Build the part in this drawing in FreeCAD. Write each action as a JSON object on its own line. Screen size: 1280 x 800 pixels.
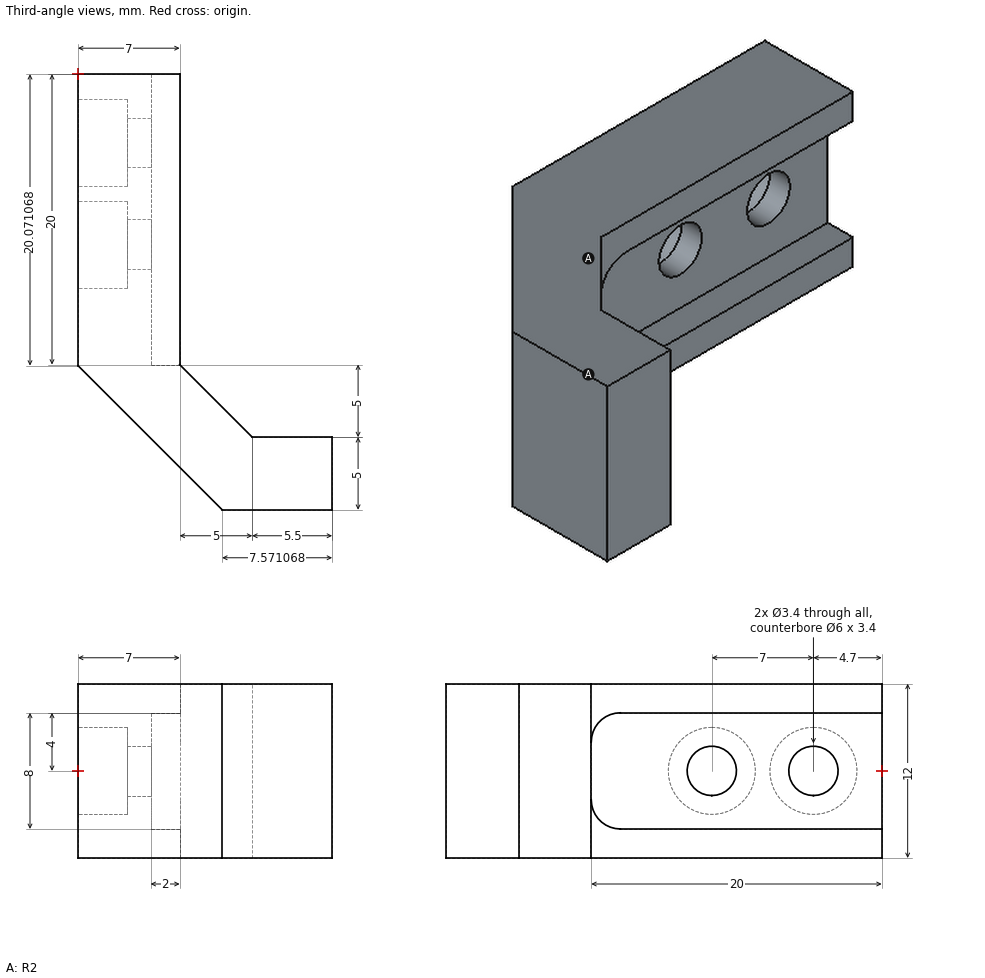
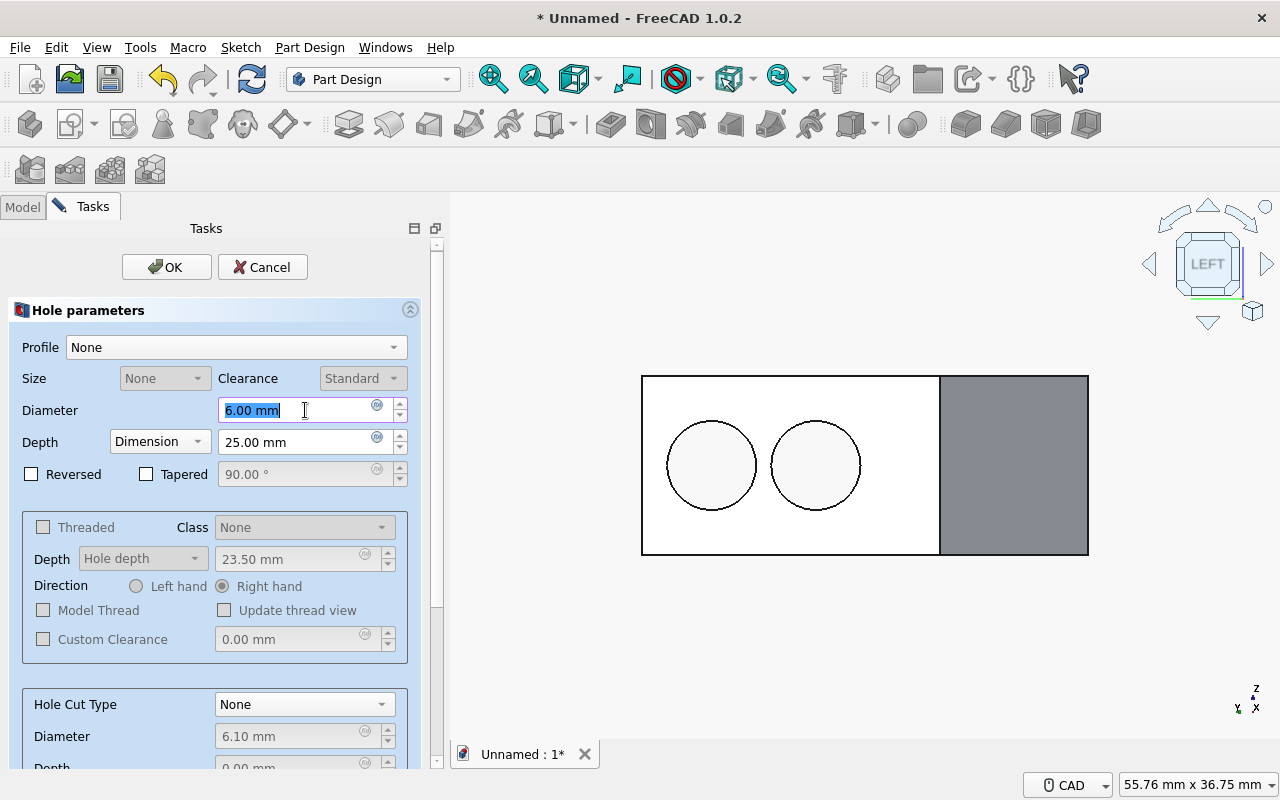
{"action": "type", "text": "3.4"}
{"action": "key", "text": "Tab"}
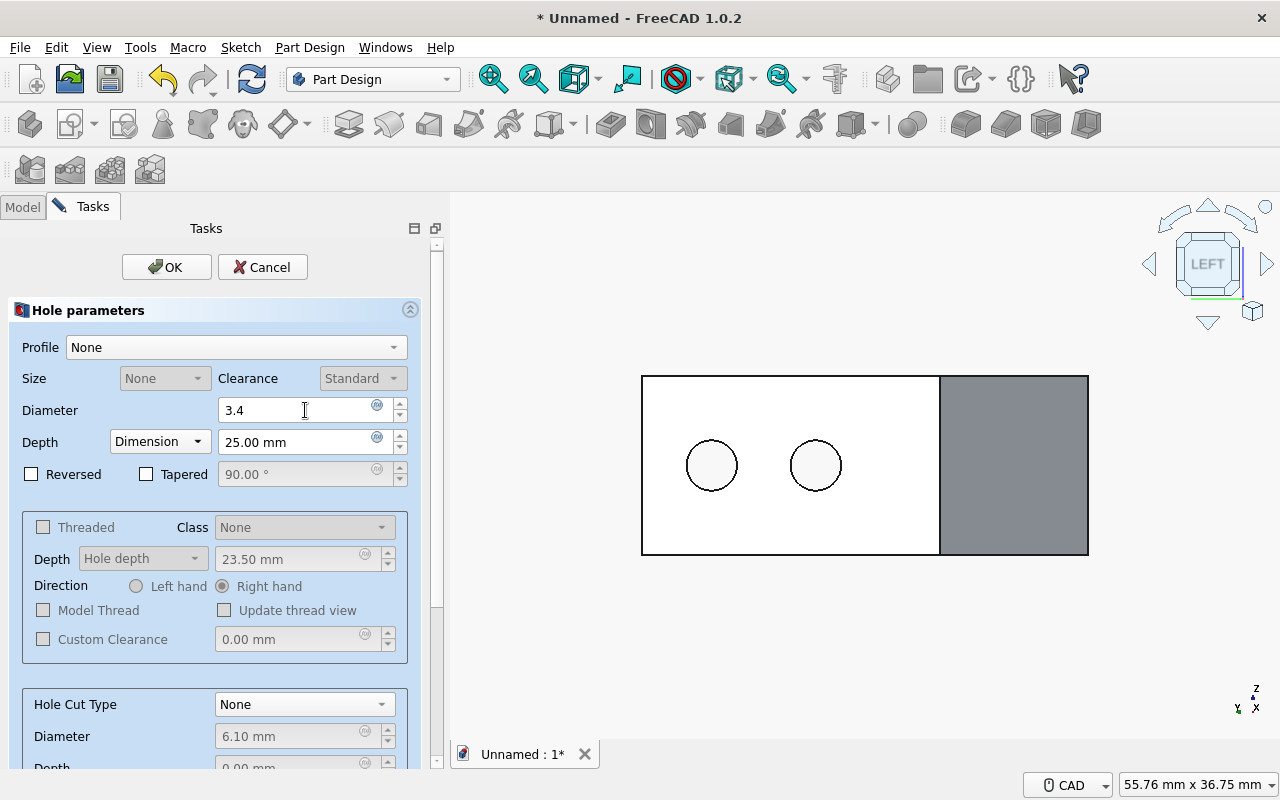
{"action": "left_click", "coordinate": [161, 442]}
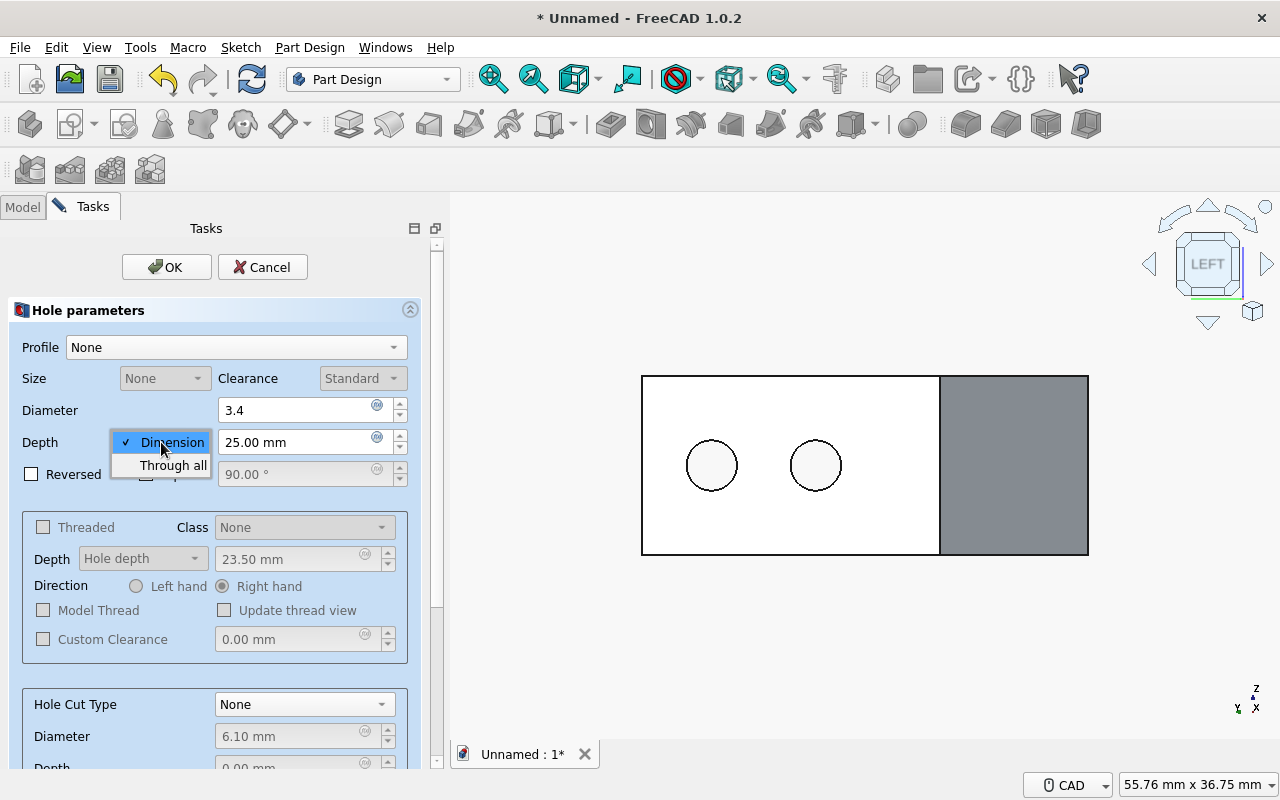
{"action": "left_click", "coordinate": [160, 466]}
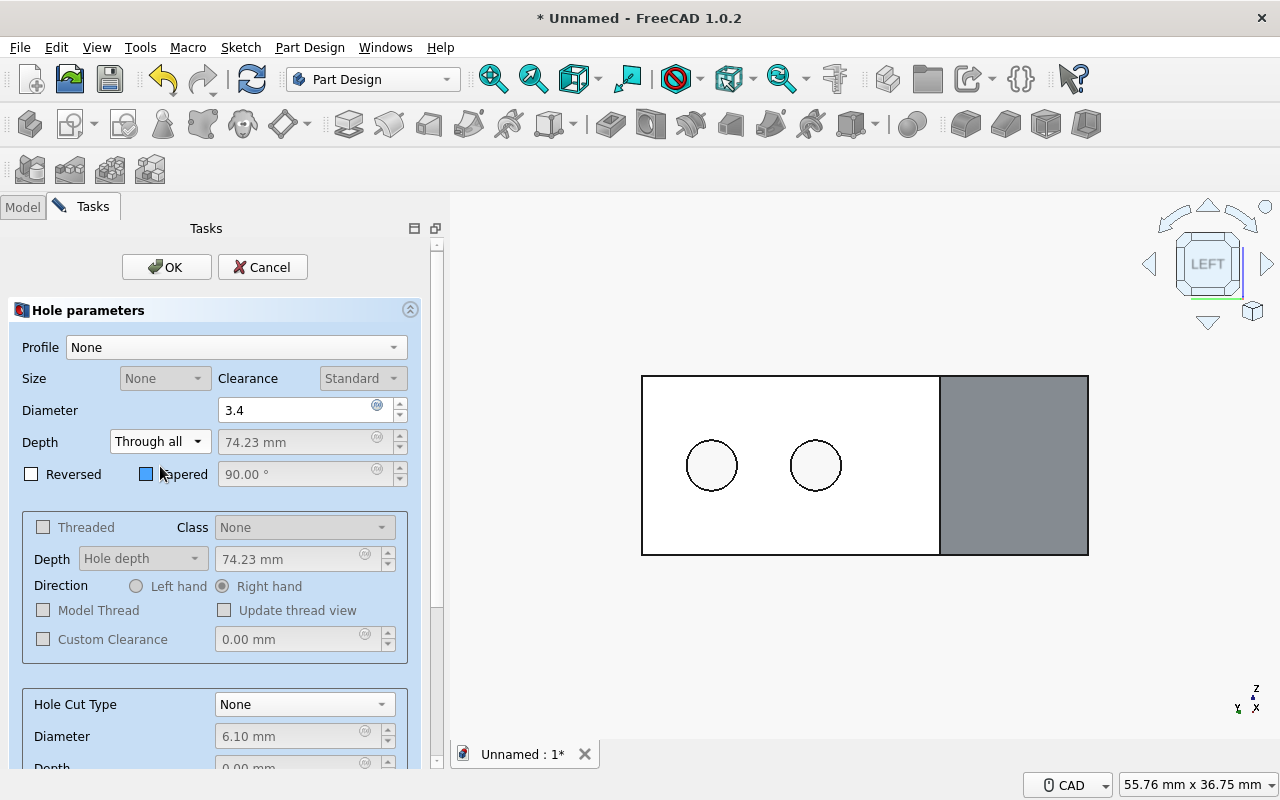
{"action": "left_click", "coordinate": [306, 704]}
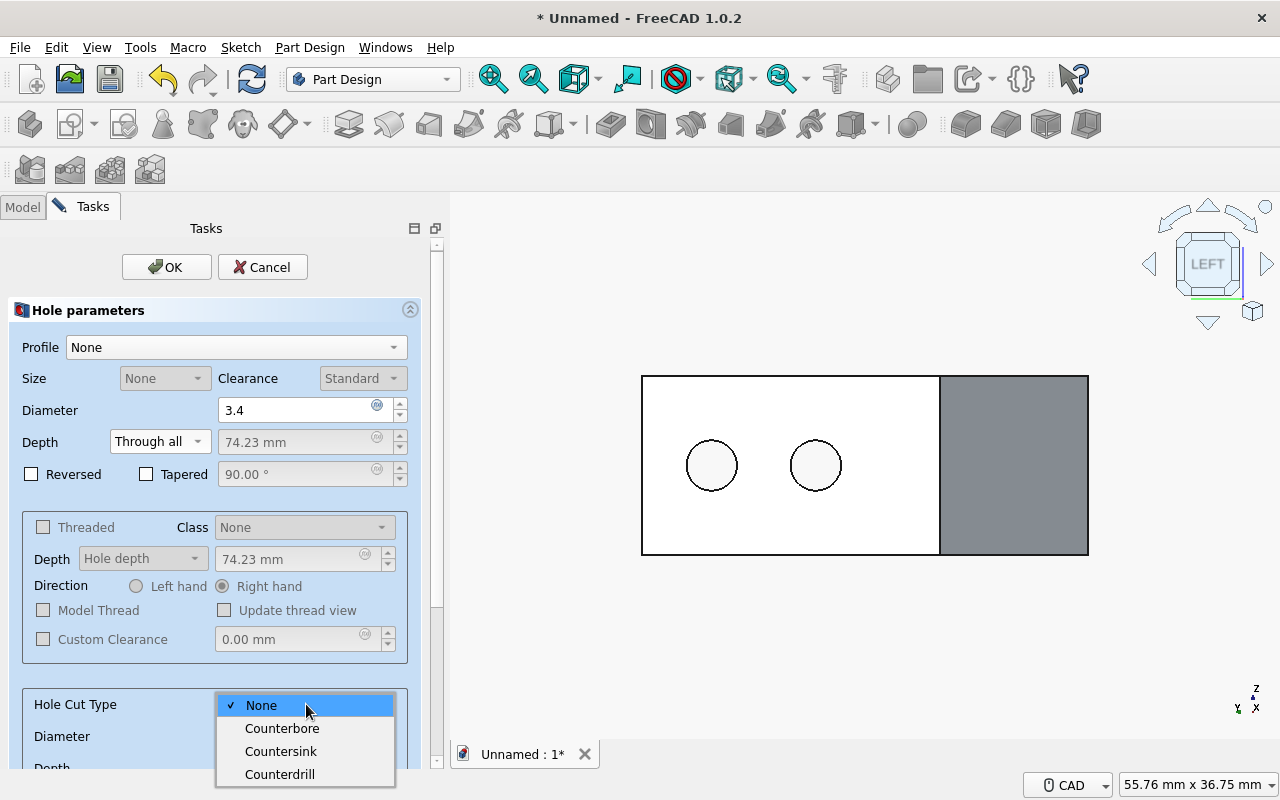
{"action": "left_click", "coordinate": [304, 728]}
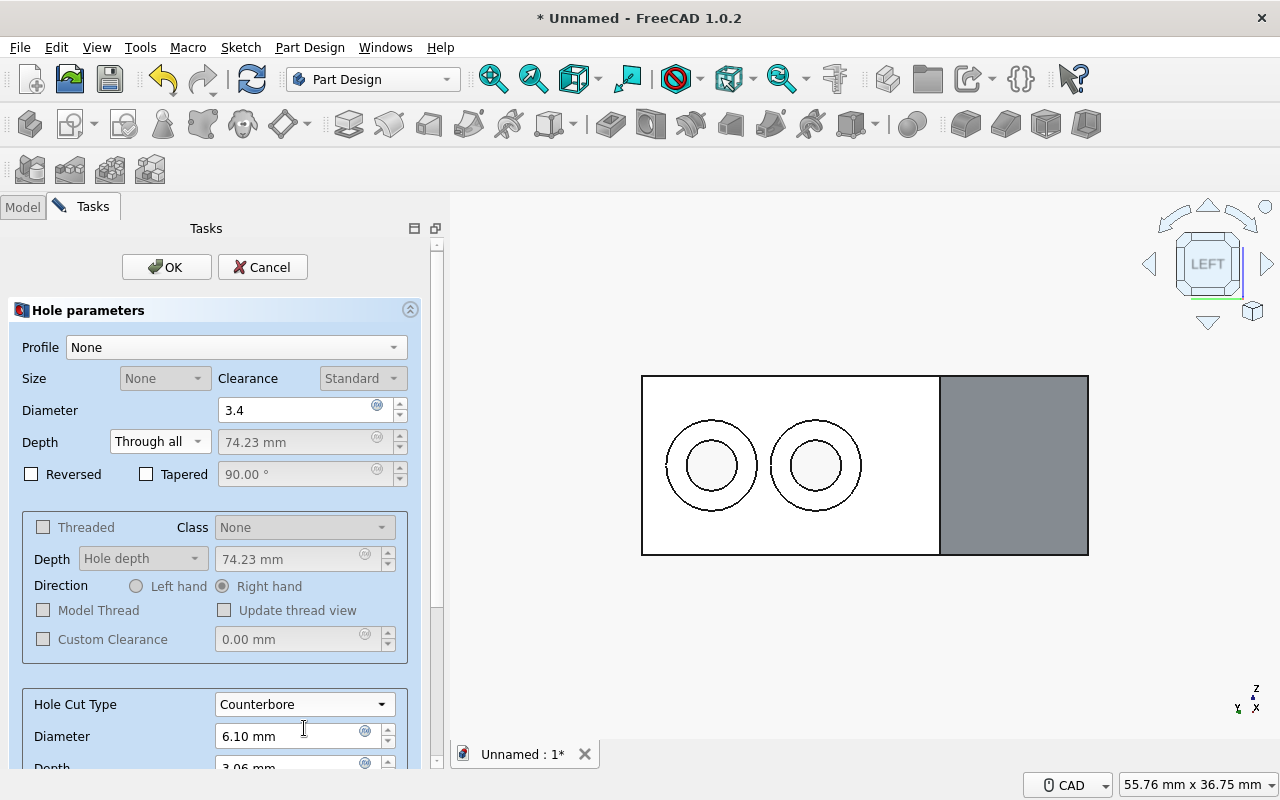
{"action": "triple_click", "coordinate": [298, 736]}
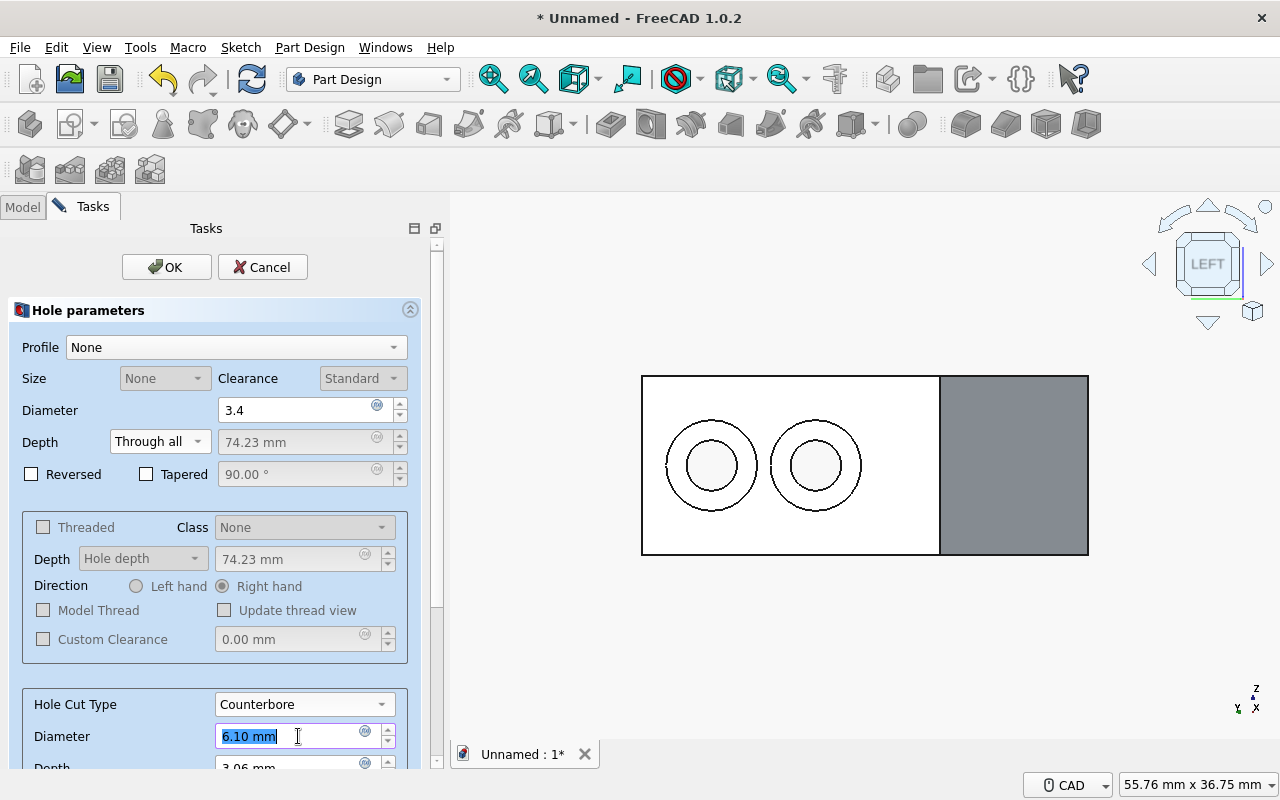
{"action": "type", "text": "6"}
{"action": "key", "text": "Tab"}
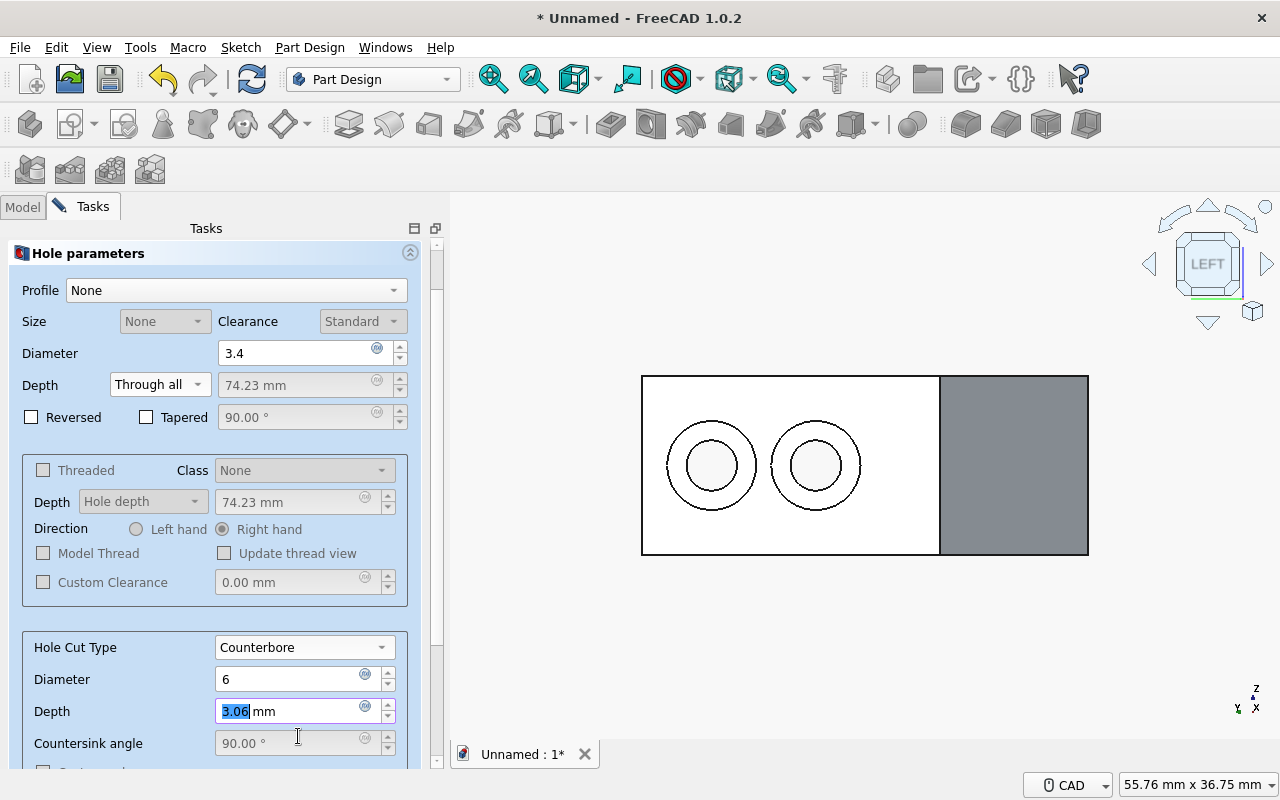
{"action": "type", "text": "3.4"}
{"action": "key", "text": "Tab"}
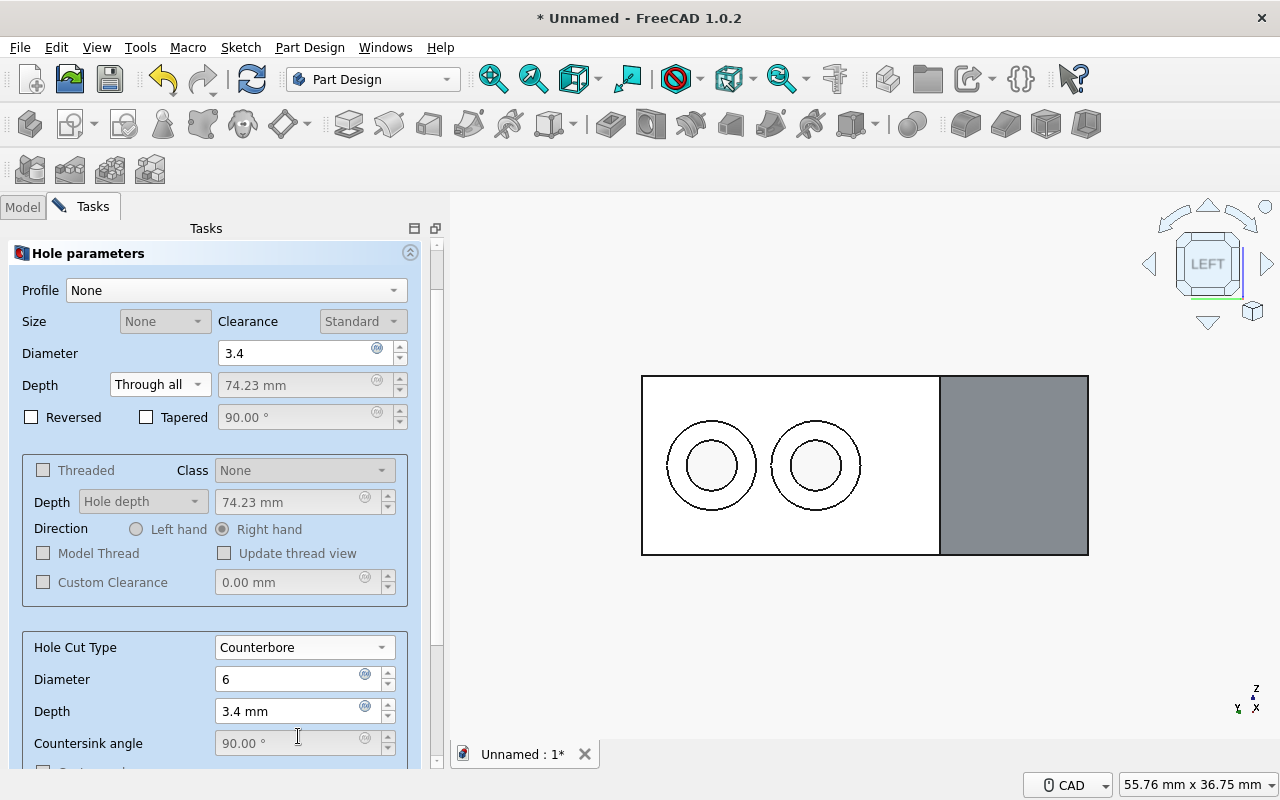
{"action": "scroll", "coordinate": [437, 503], "scroll_direction": "up", "scroll_amount": 2}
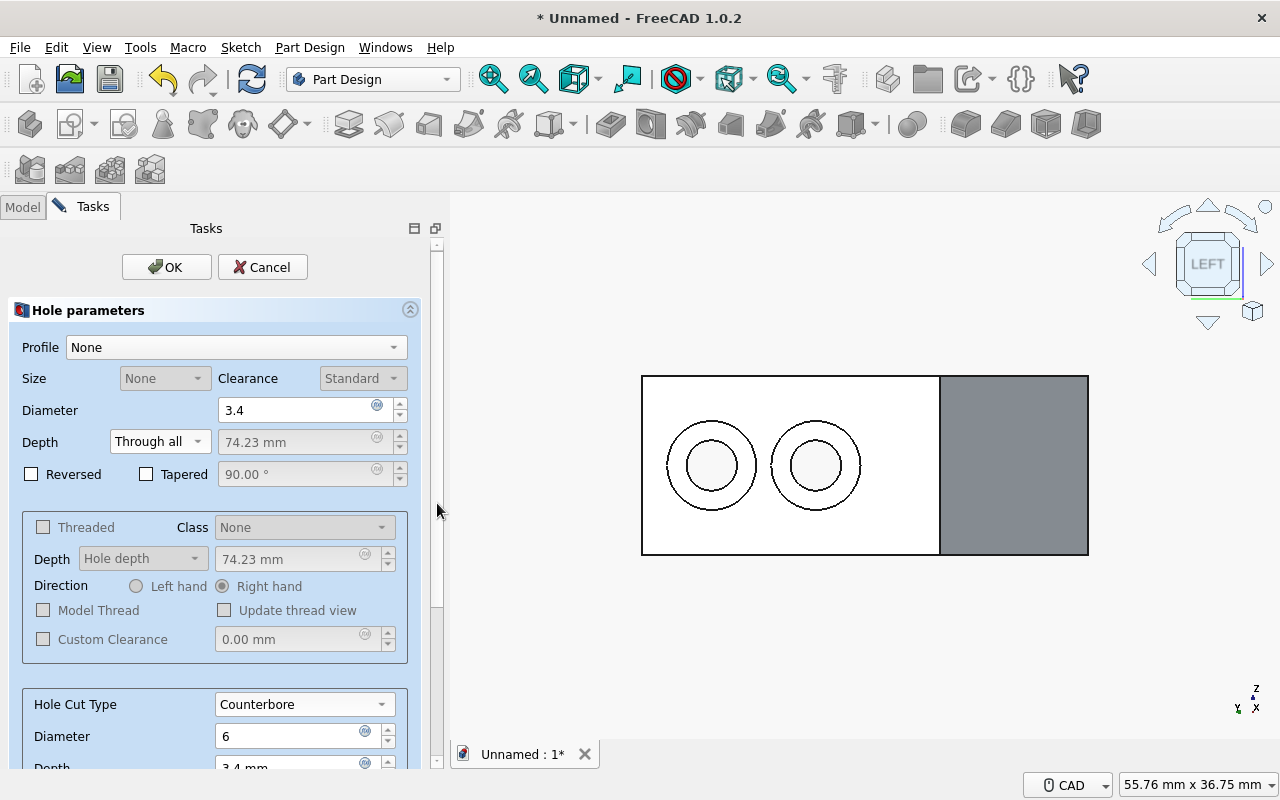
{"action": "left_click", "coordinate": [167, 267]}